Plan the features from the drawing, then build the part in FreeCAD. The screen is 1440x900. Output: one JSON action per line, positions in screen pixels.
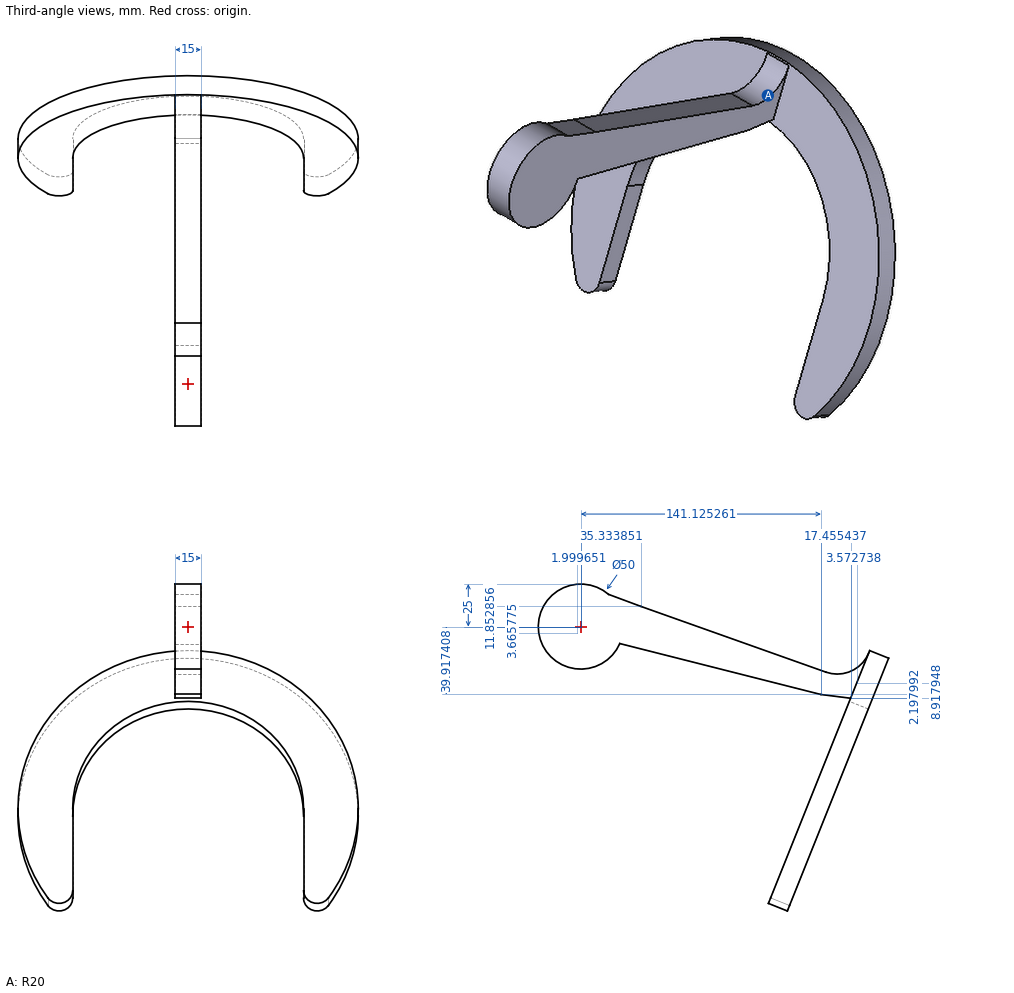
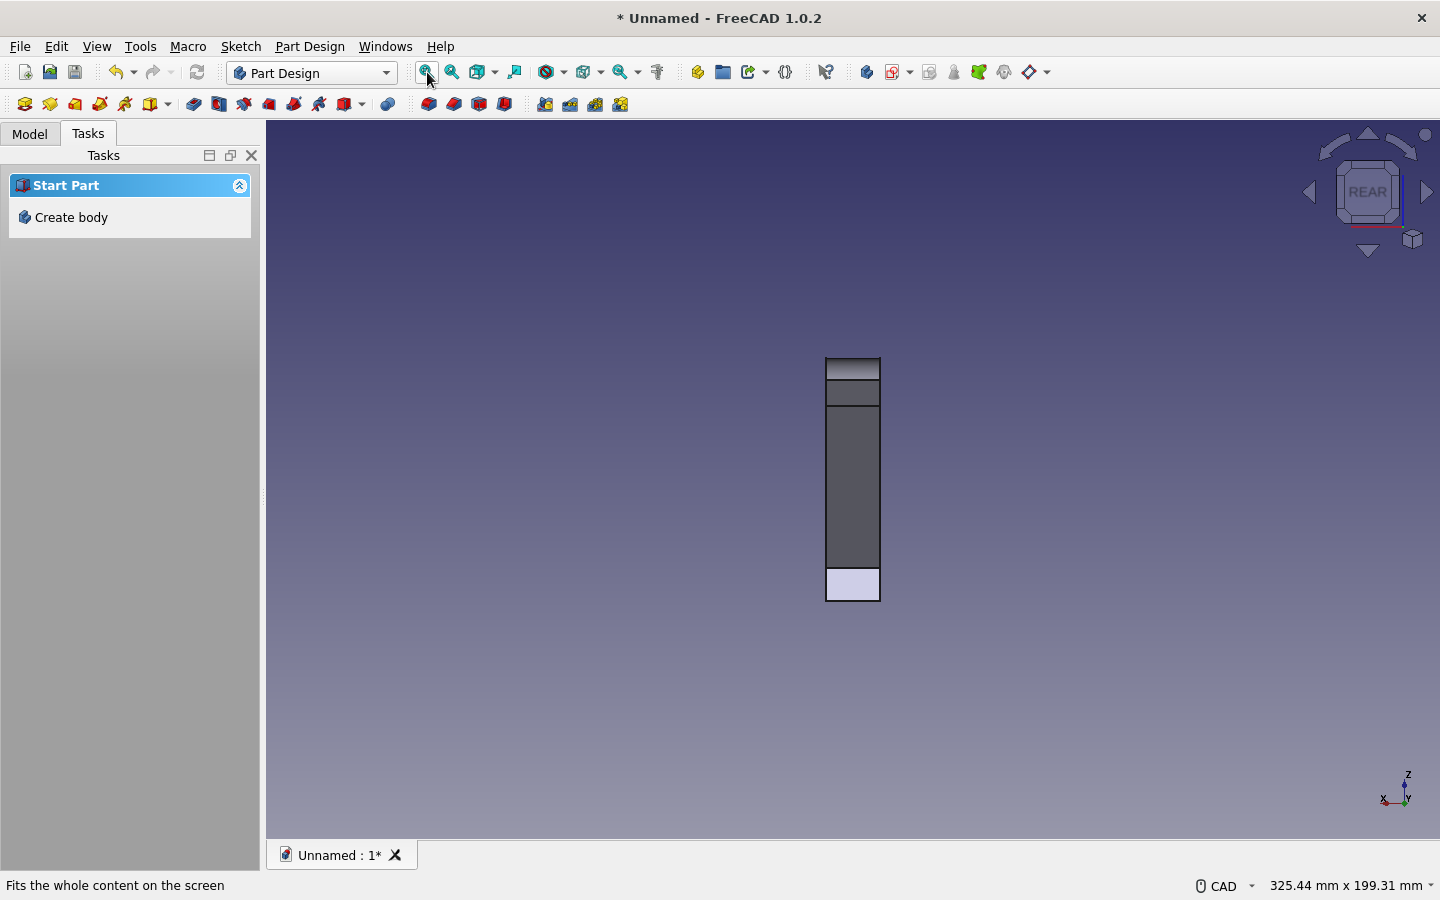
{"action": "left_click", "coordinate": [845, 583]}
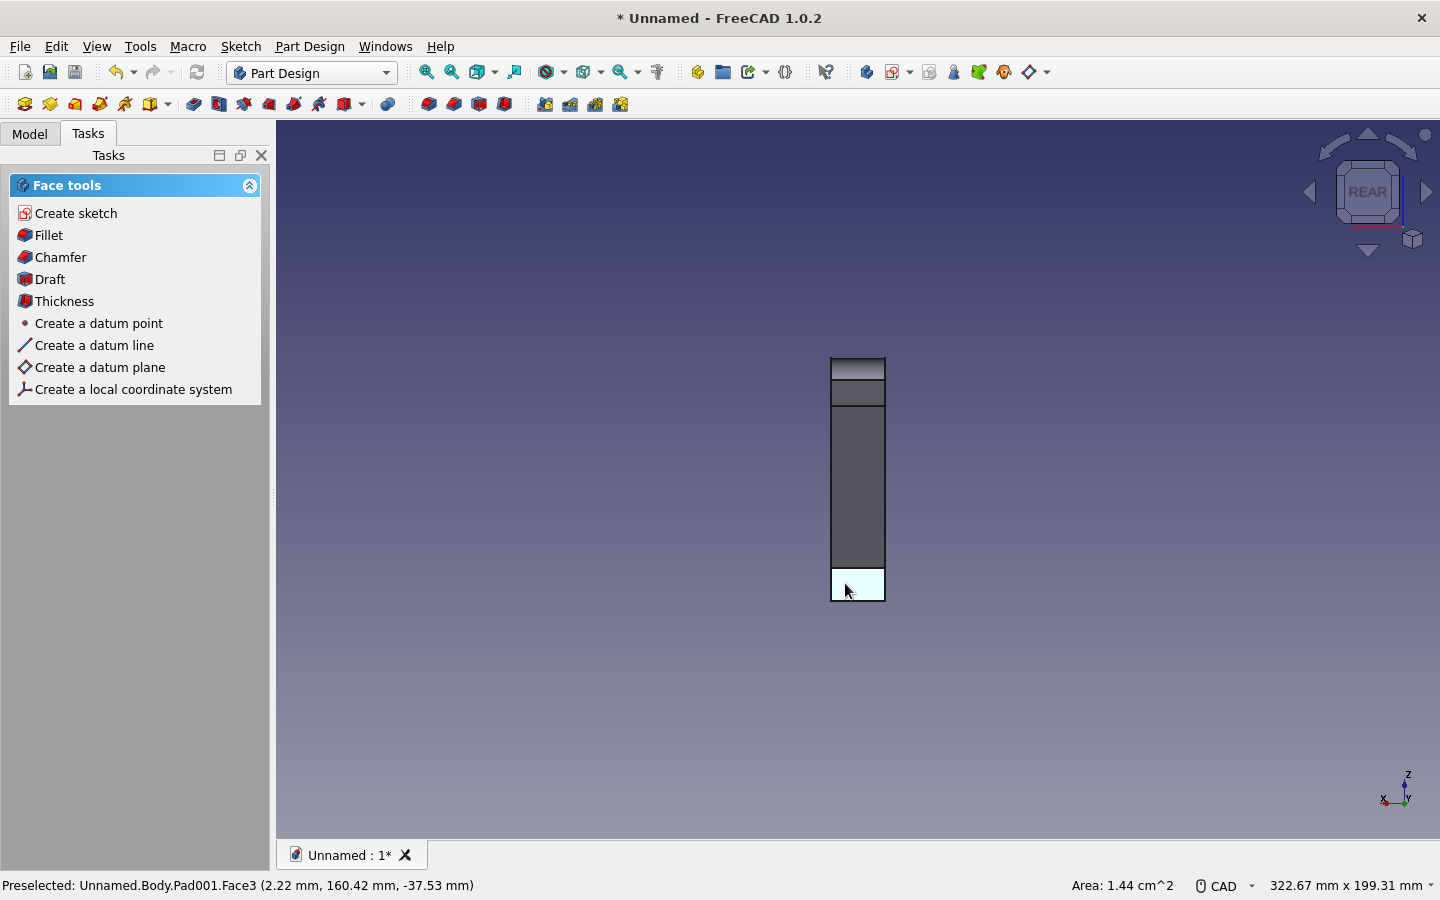
{"action": "left_click", "coordinate": [892, 72]}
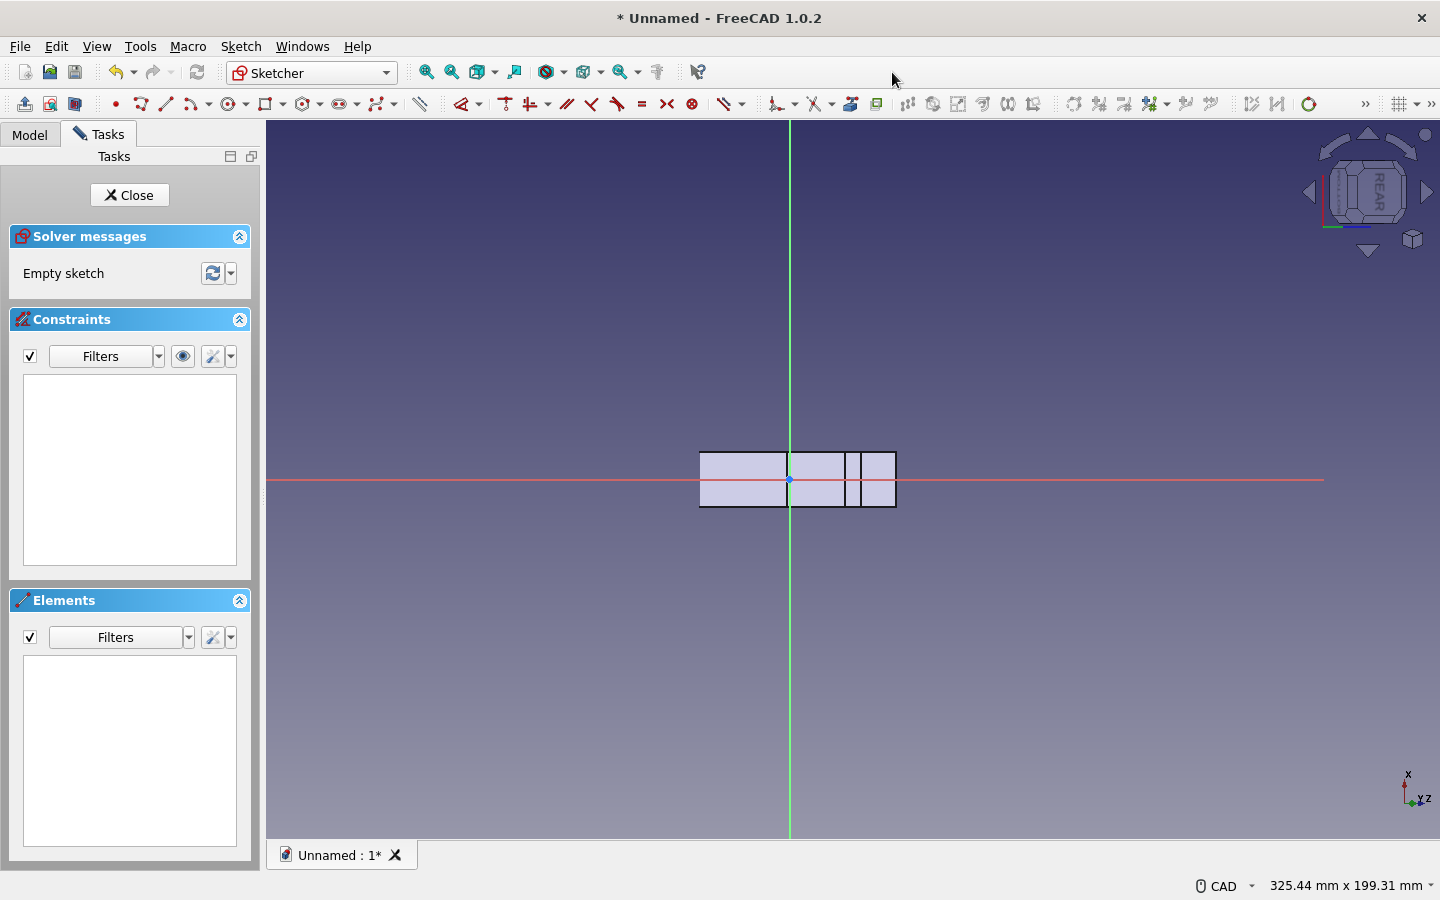
{"action": "left_click", "coordinate": [166, 104]}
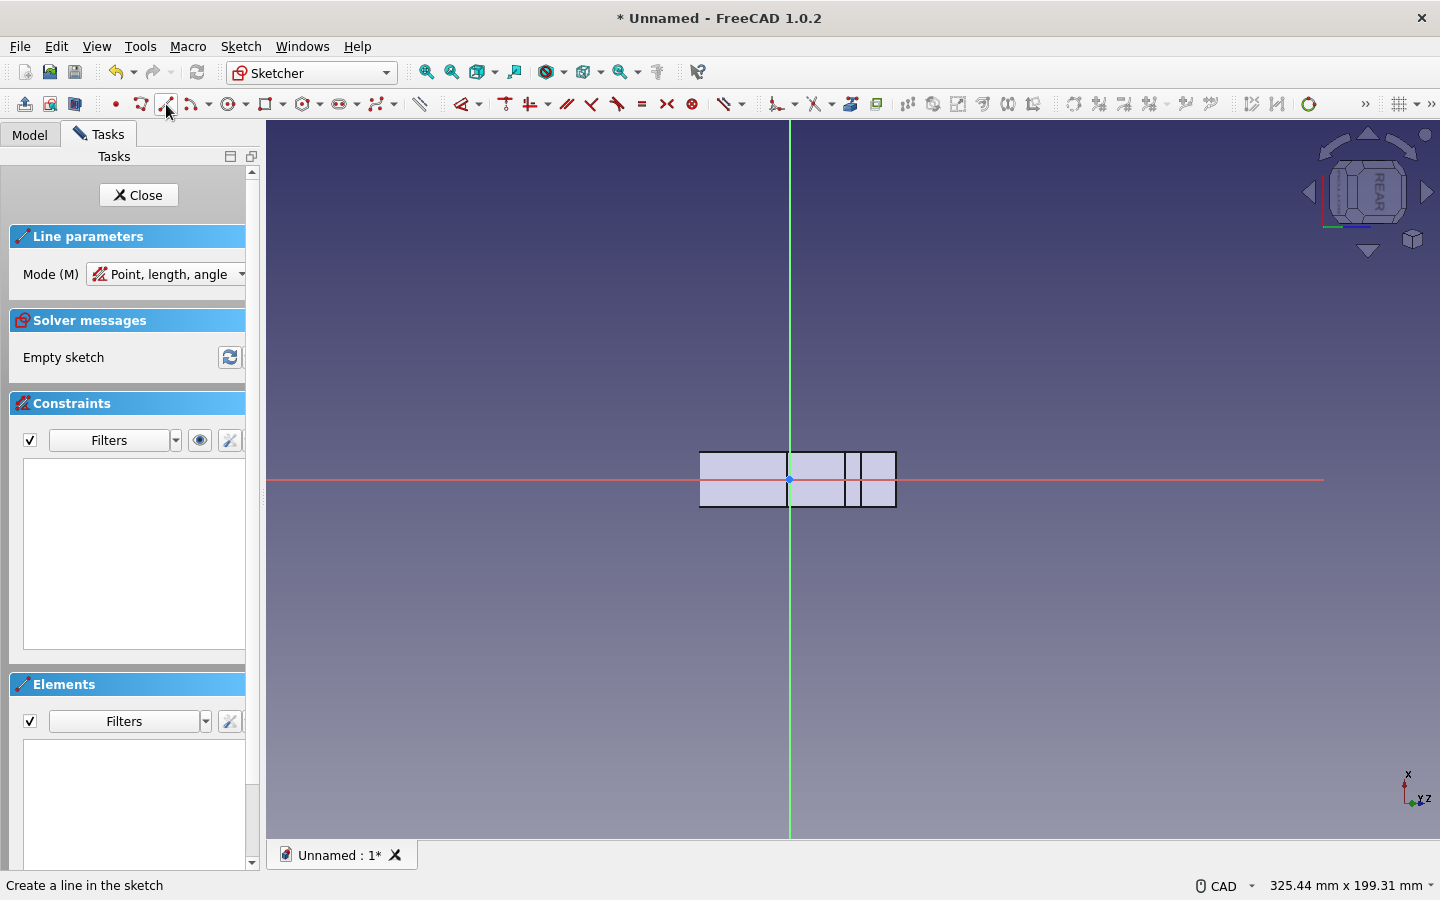
{"action": "left_click", "coordinate": [422, 235]}
{"action": "left_click", "coordinate": [609, 235]}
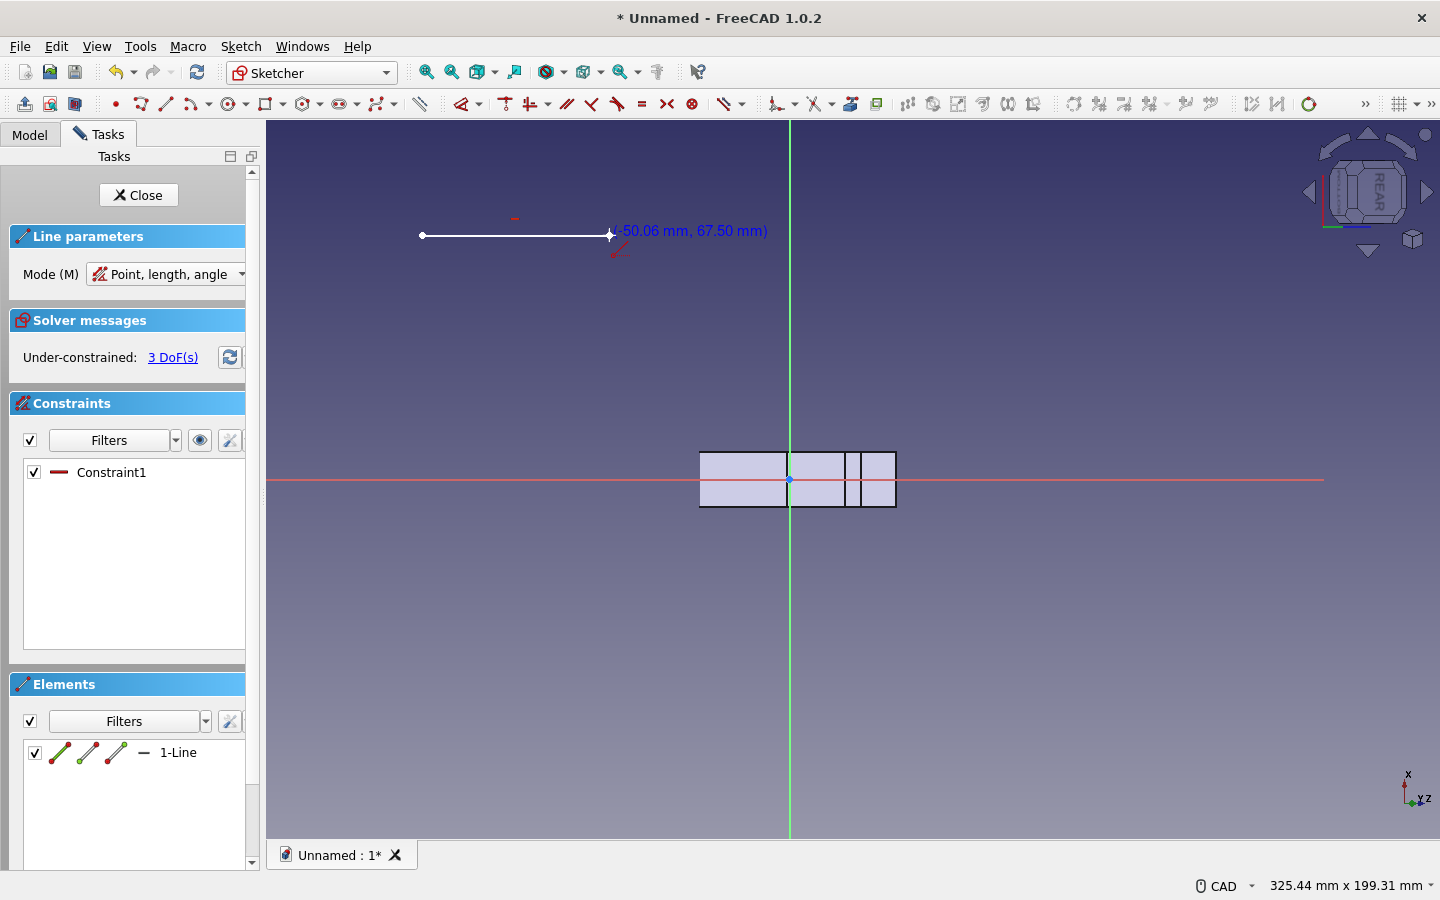
{"action": "left_click", "coordinate": [609, 724]}
{"action": "left_click", "coordinate": [422, 724]}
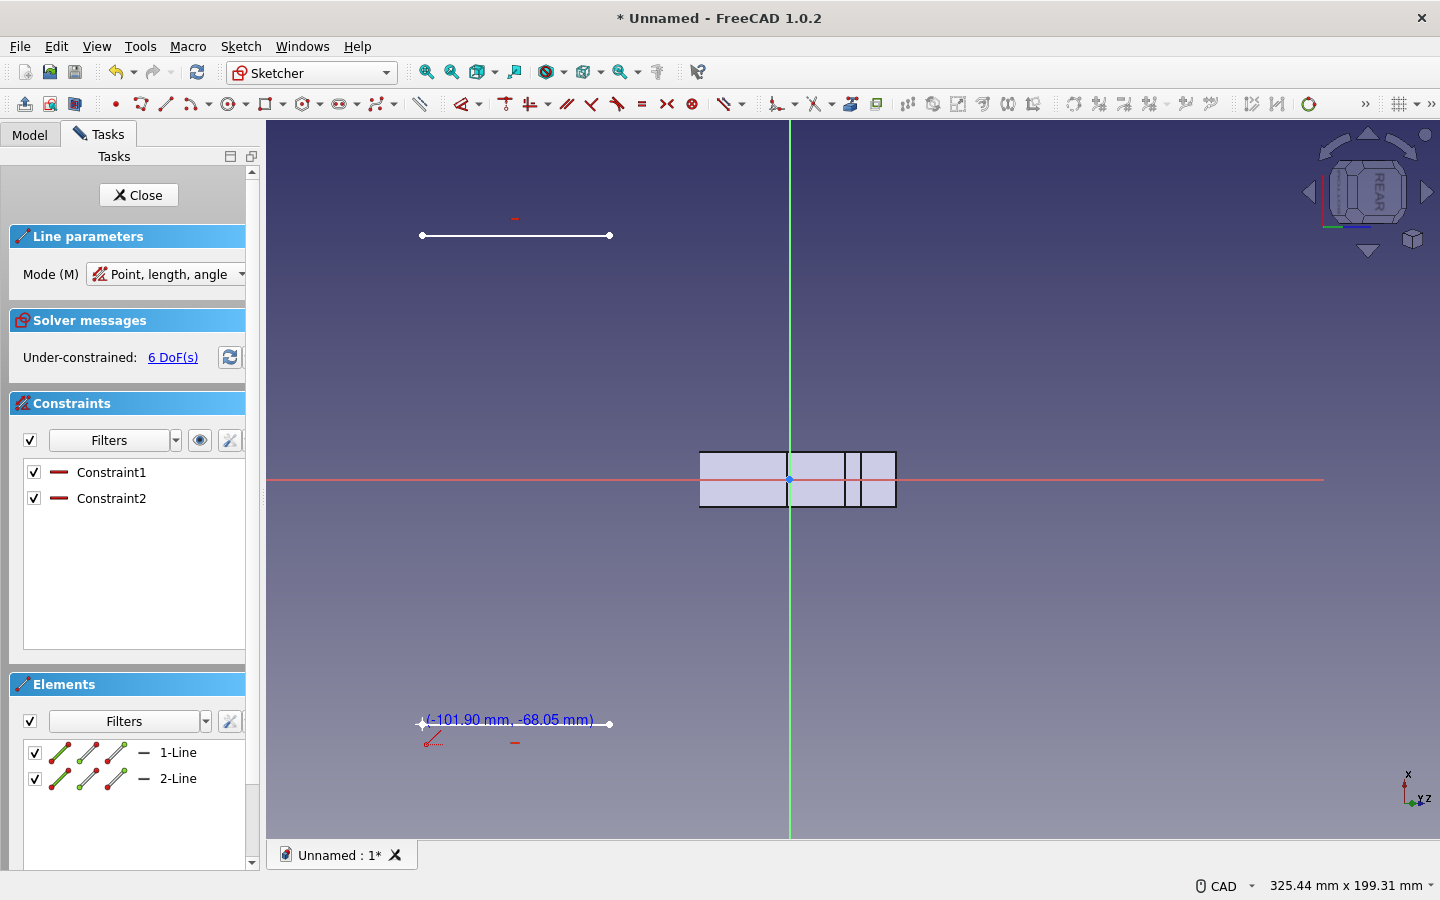
{"action": "left_click", "coordinate": [208, 104]}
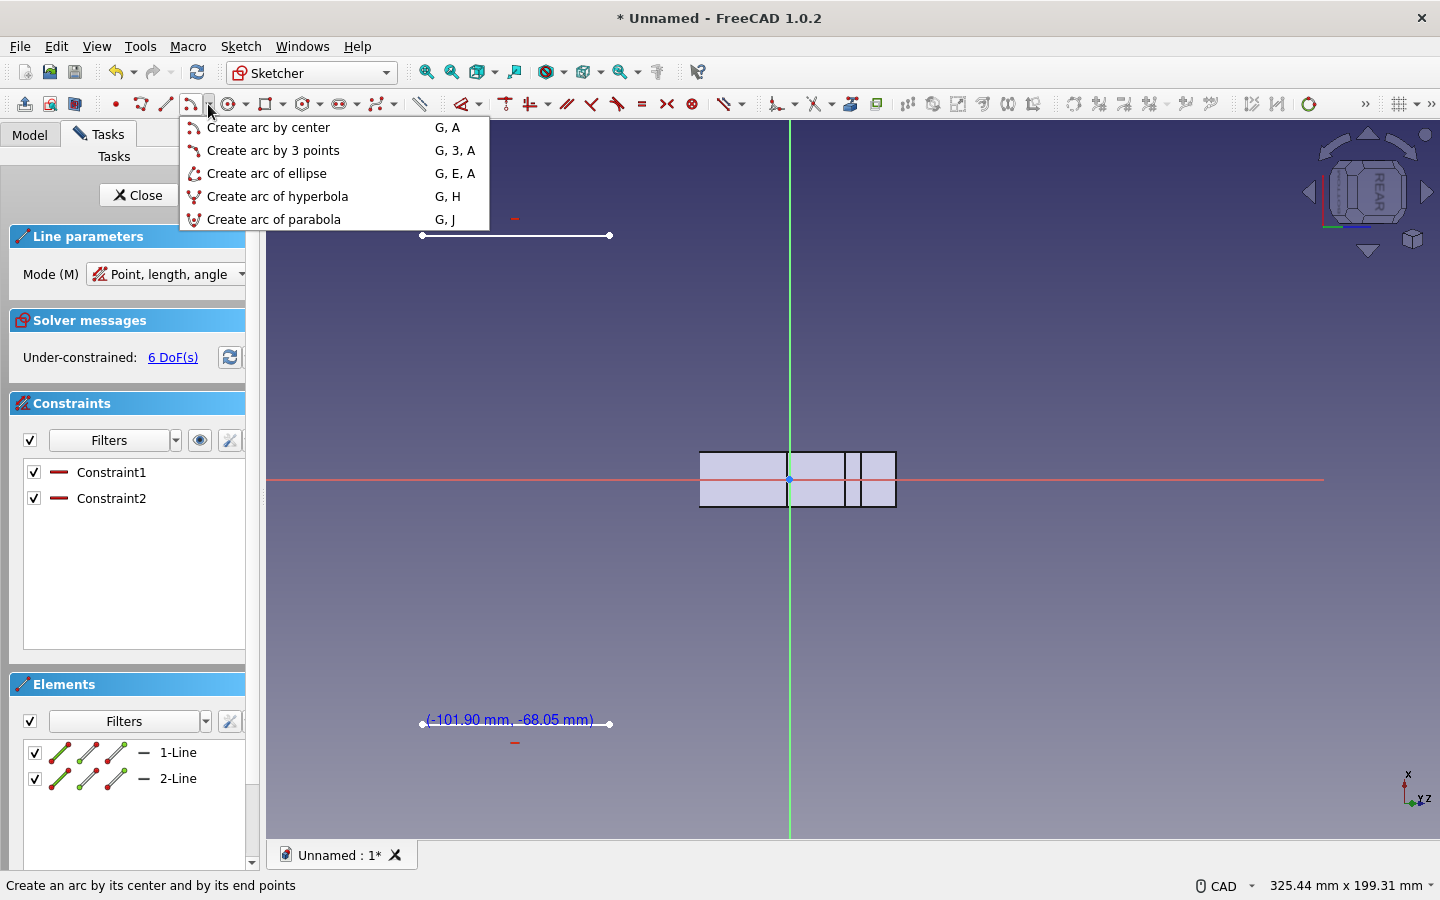
{"action": "left_click", "coordinate": [334, 150]}